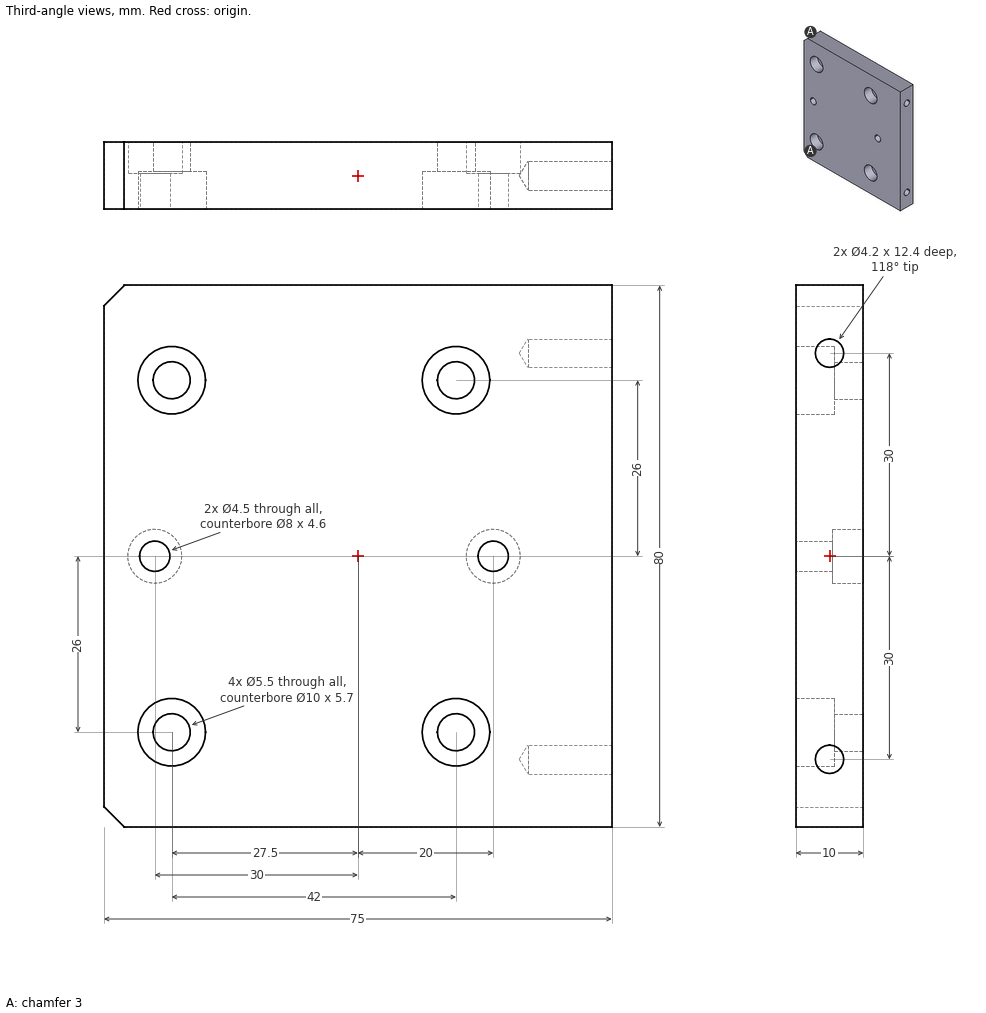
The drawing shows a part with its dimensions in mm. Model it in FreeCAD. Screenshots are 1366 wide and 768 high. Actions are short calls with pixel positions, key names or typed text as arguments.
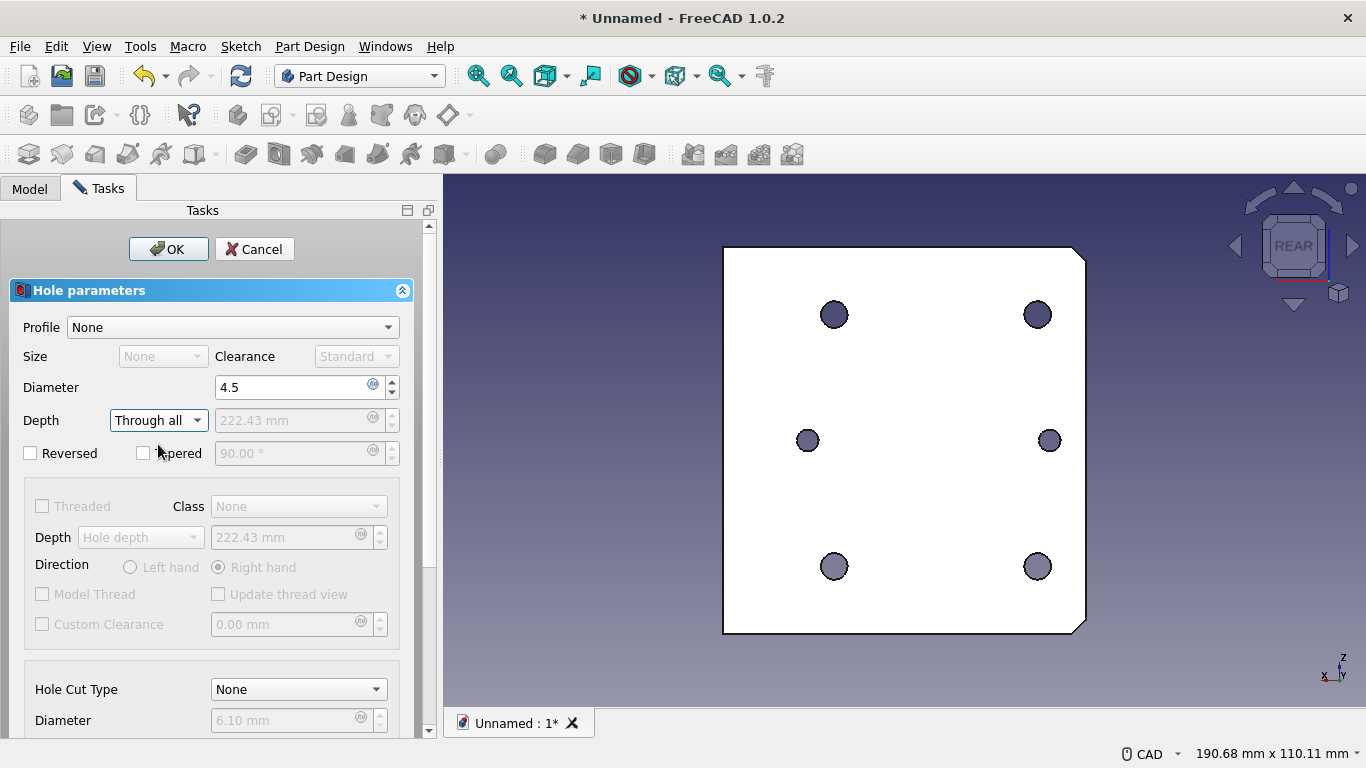
click(300, 690)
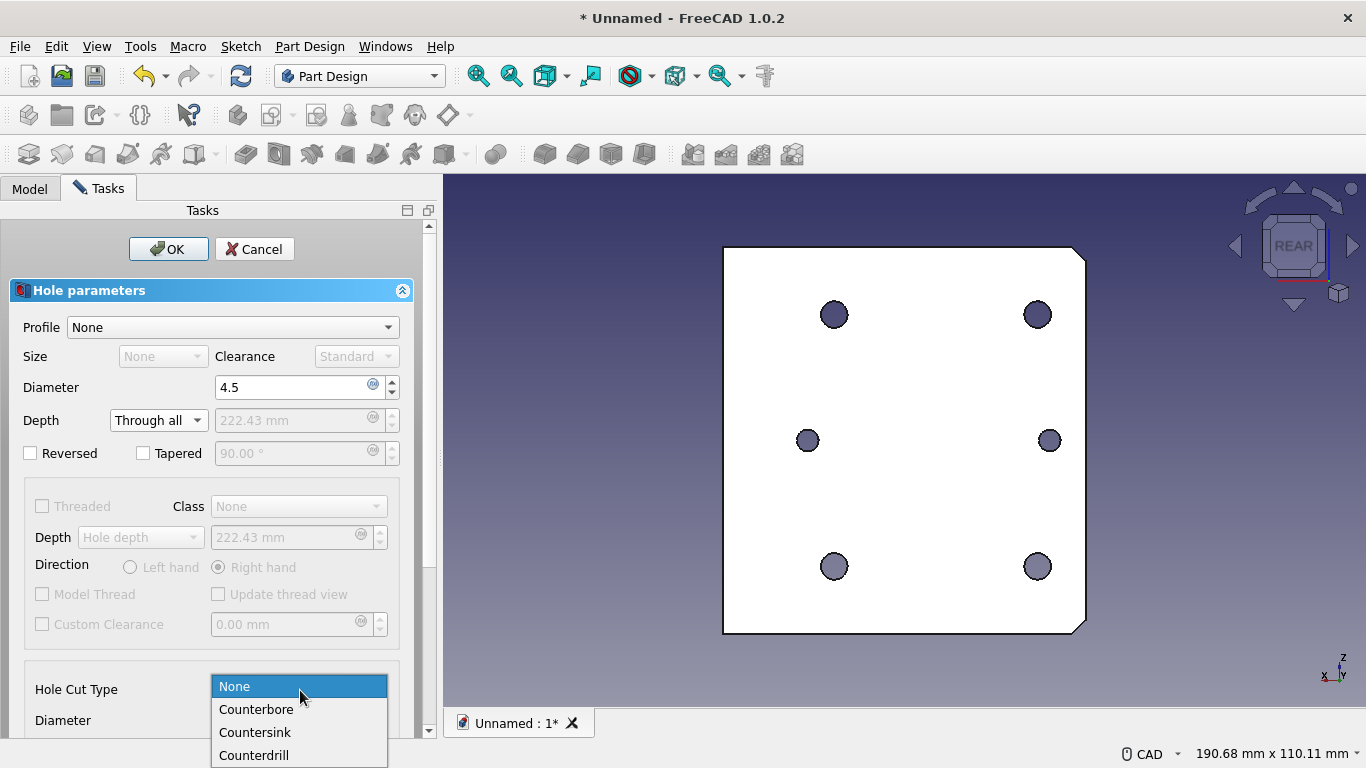
click(298, 710)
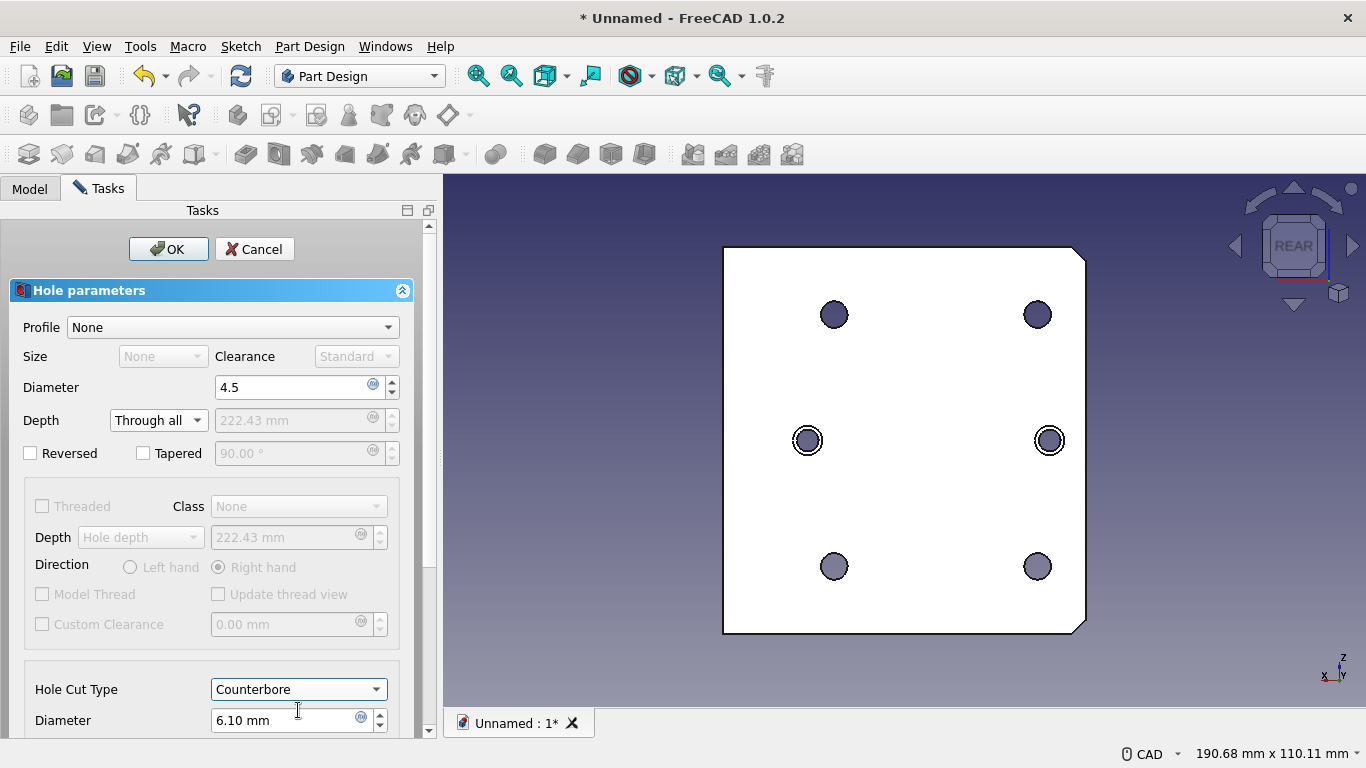
triple_click(292, 720)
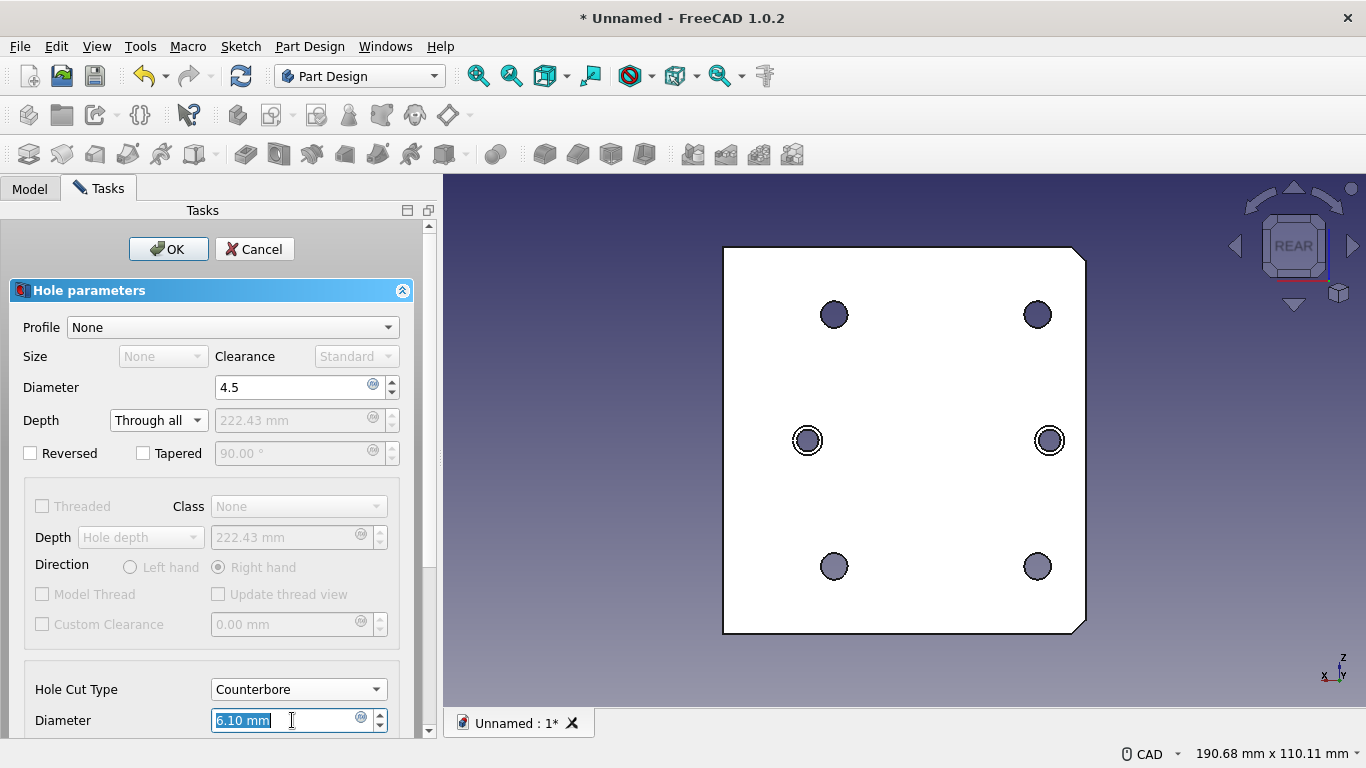
text(8)
key(Tab)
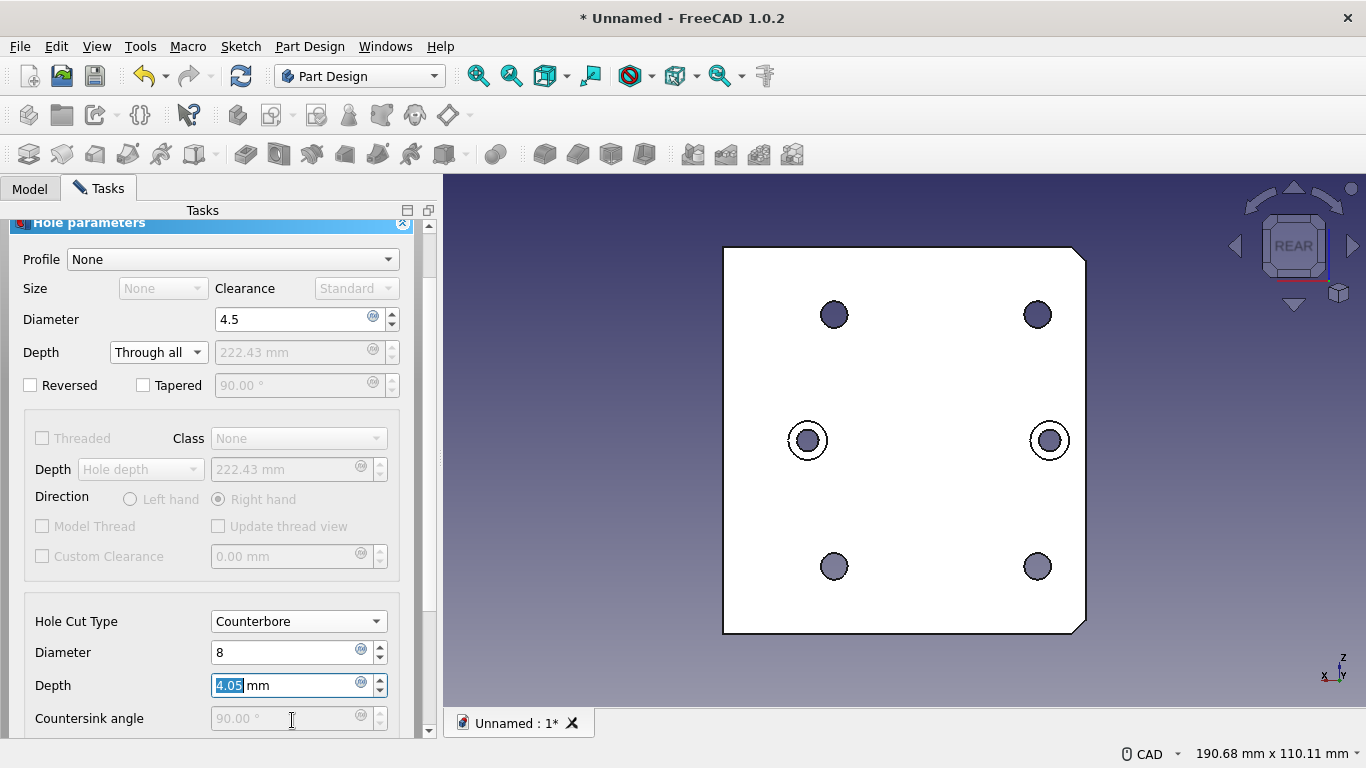
text(4.6)
key(Tab)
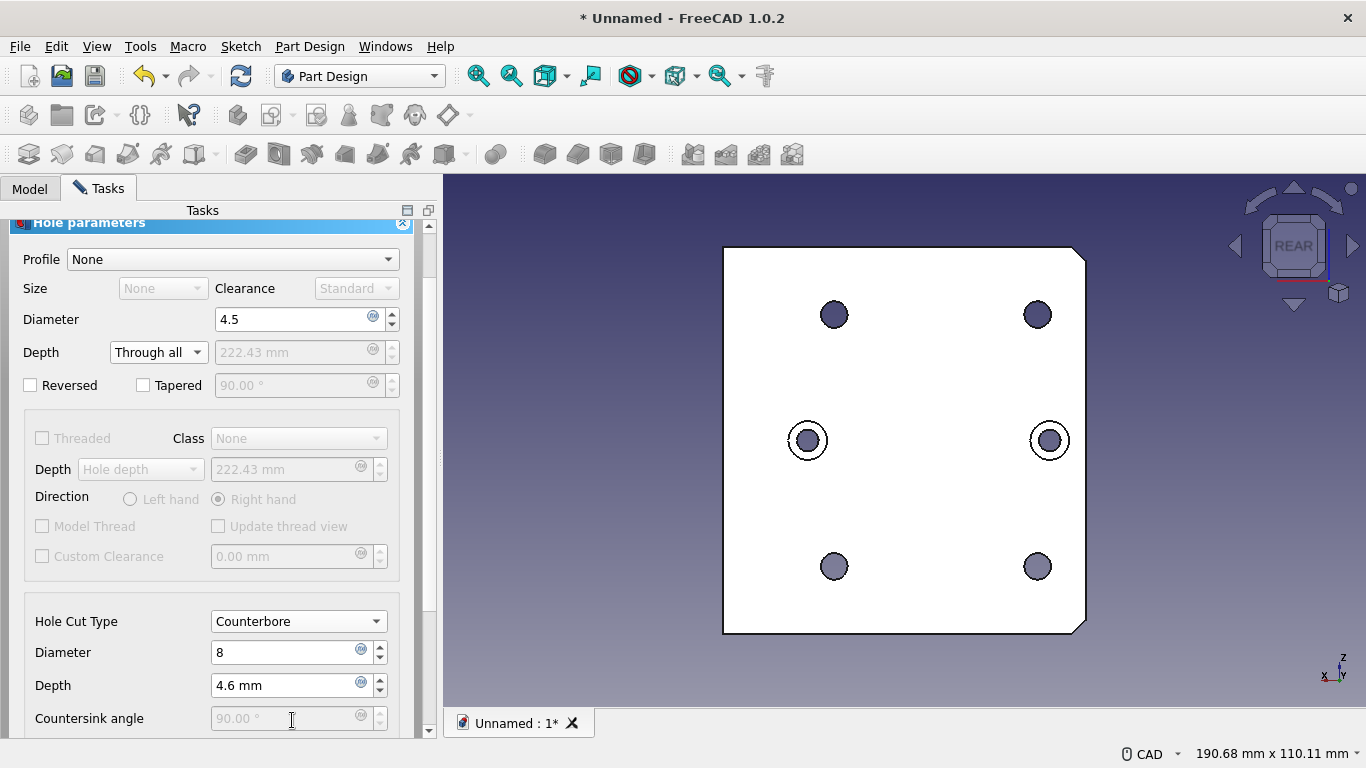
scroll(429, 479, up, 2)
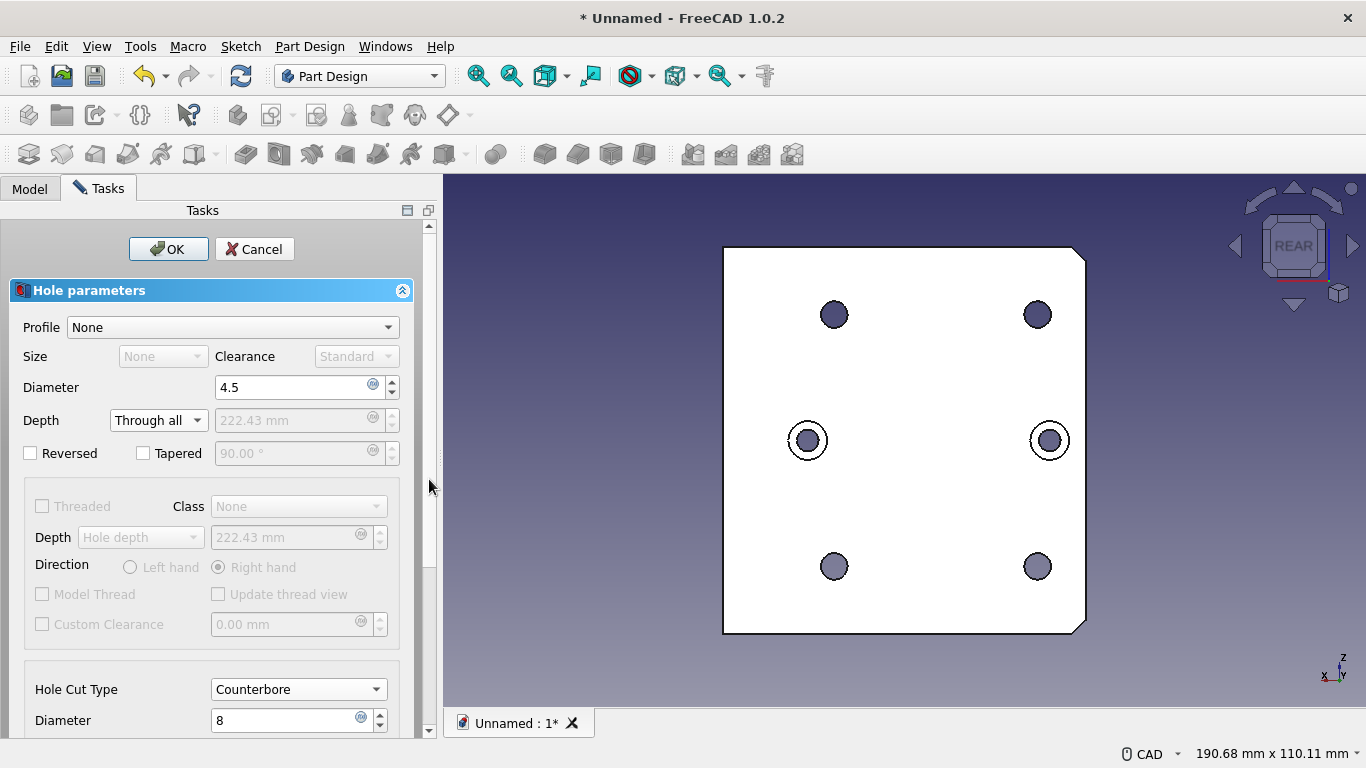
click(169, 249)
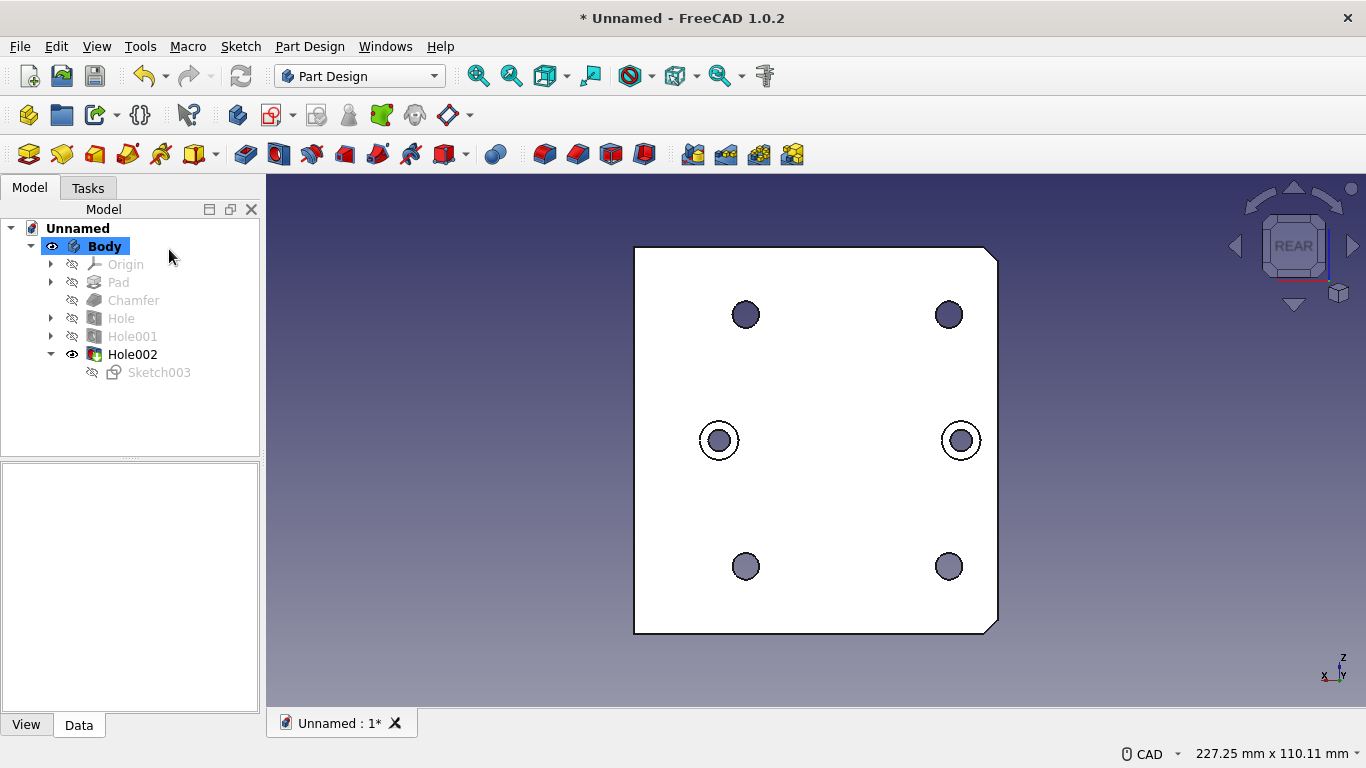
key(0)